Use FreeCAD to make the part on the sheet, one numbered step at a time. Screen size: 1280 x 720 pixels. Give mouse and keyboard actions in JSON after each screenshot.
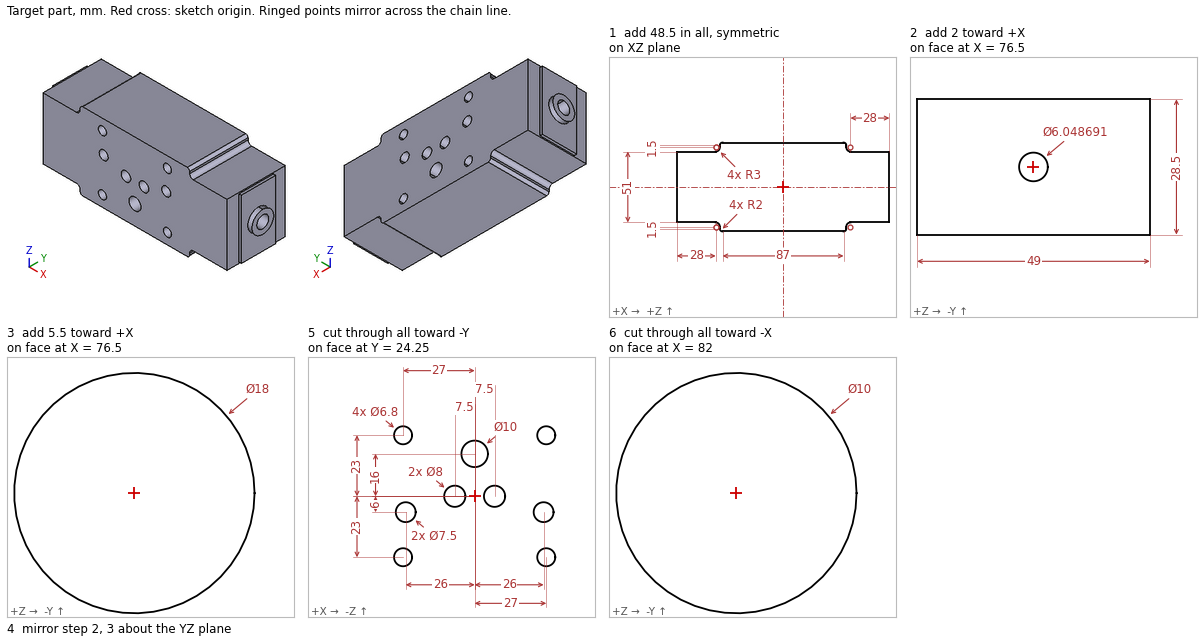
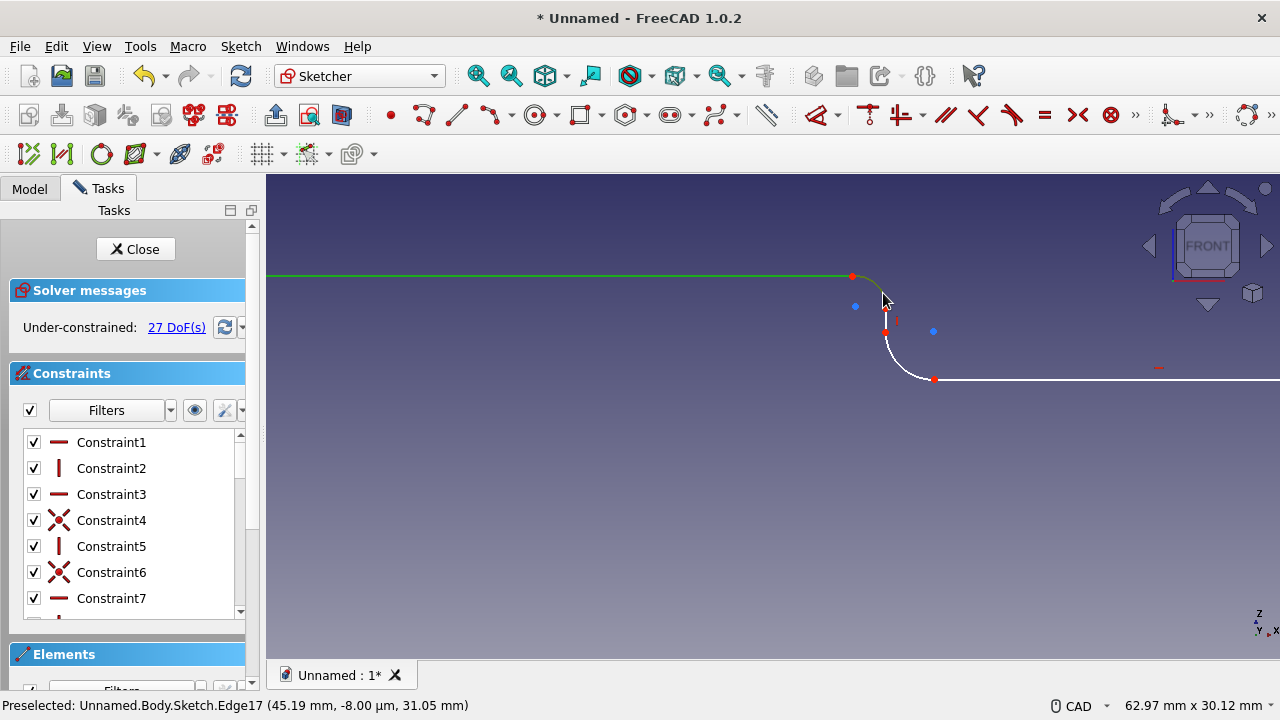
{"action": "left_click", "coordinate": [1012, 116]}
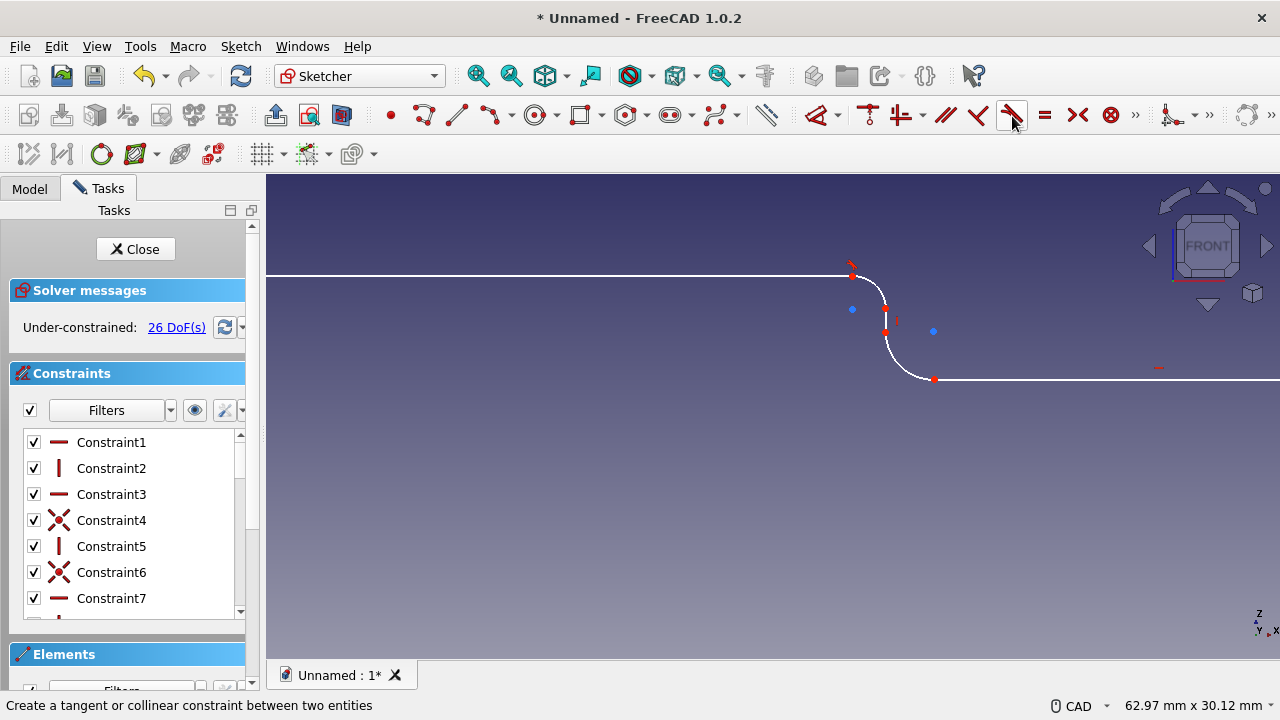
{"action": "scroll", "coordinate": [886, 318], "scroll_direction": "up", "scroll_amount": 2}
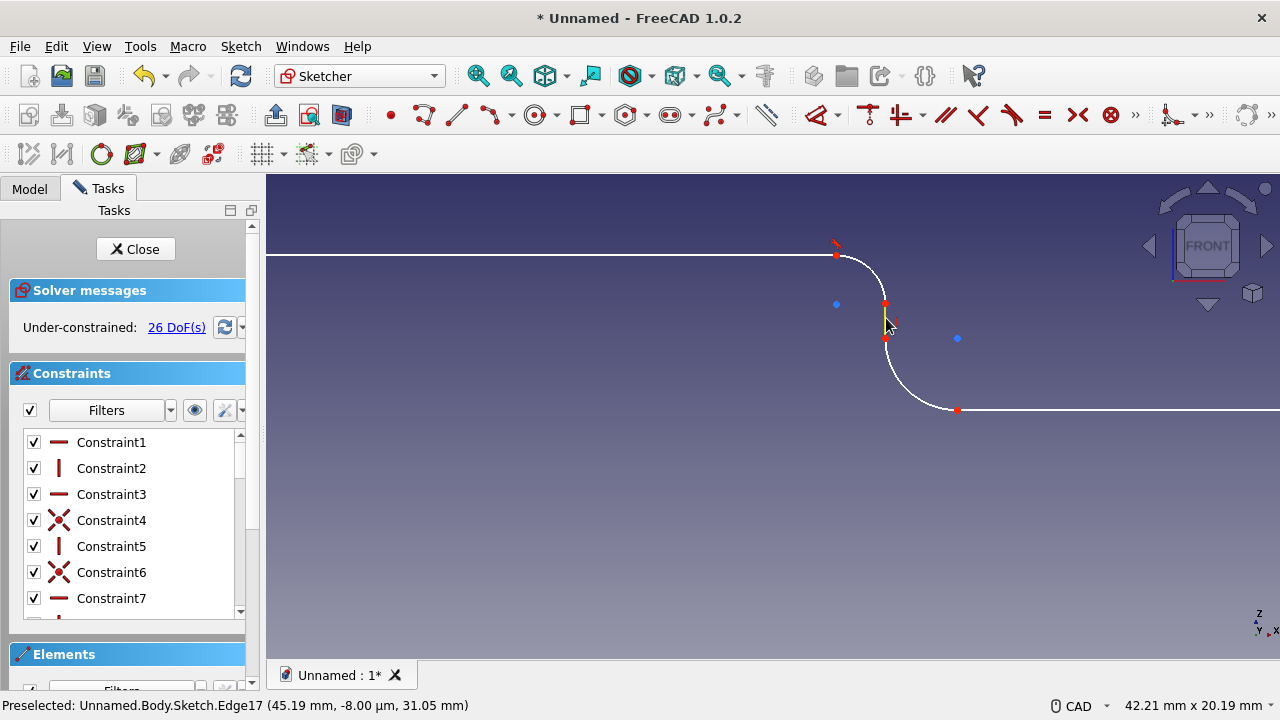
{"action": "left_click", "coordinate": [885, 318]}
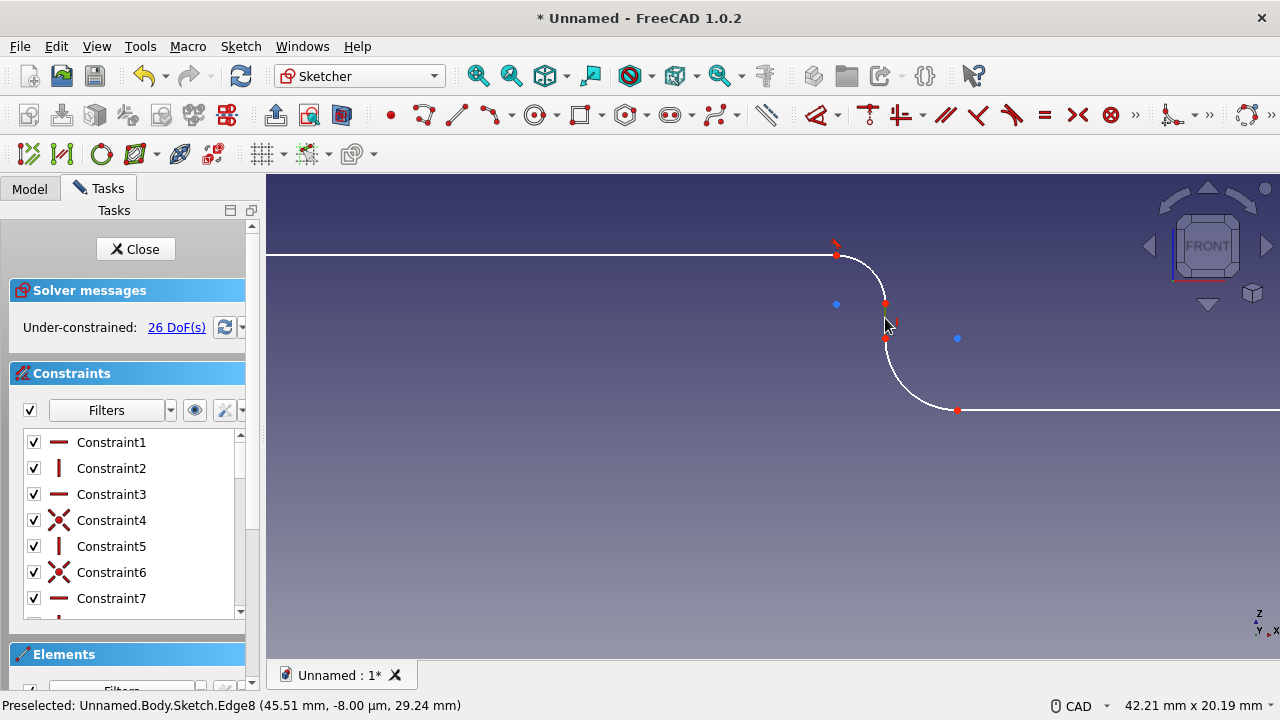
{"action": "left_click", "coordinate": [880, 282]}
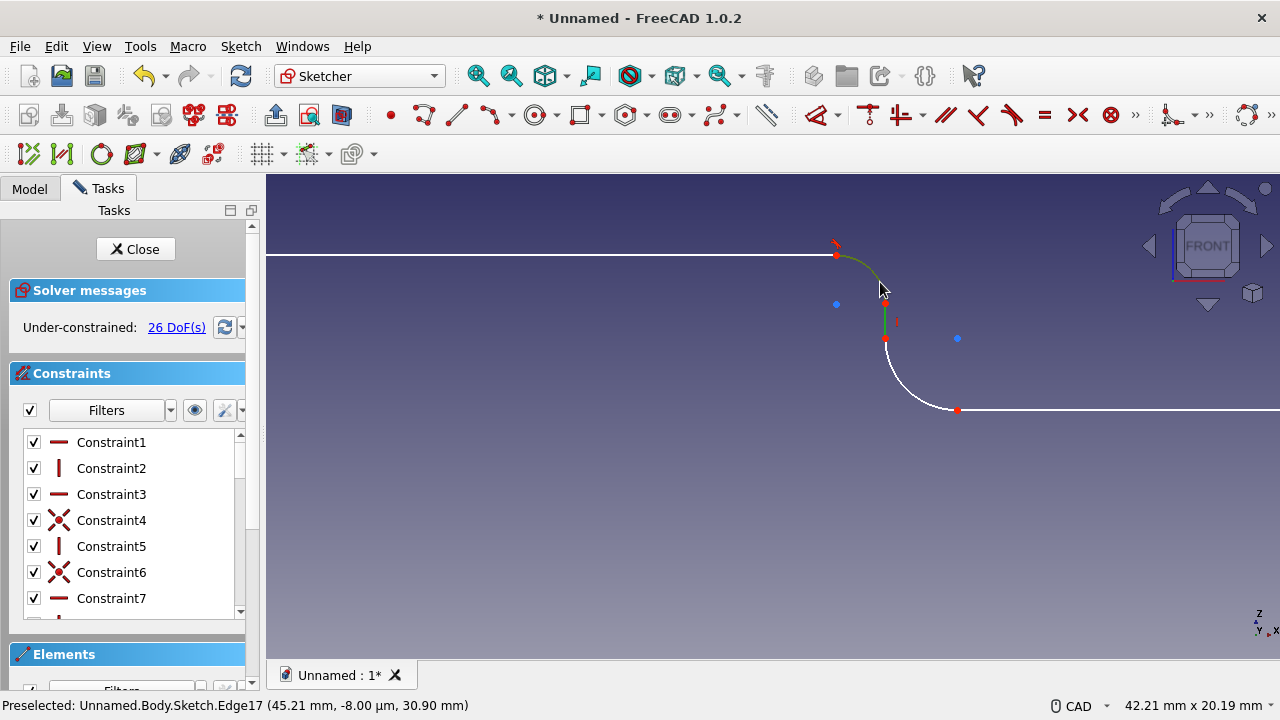
{"action": "left_click", "coordinate": [1012, 116]}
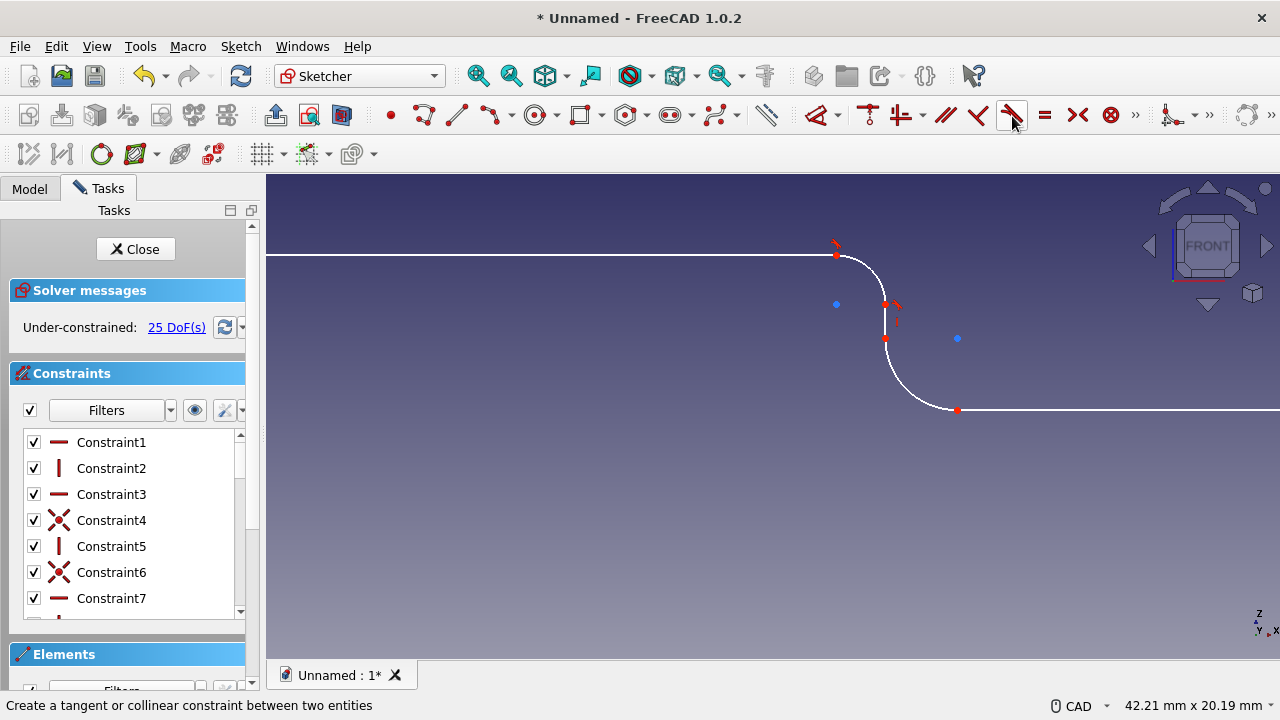
{"action": "scroll", "coordinate": [885, 315], "scroll_direction": "up", "scroll_amount": 2}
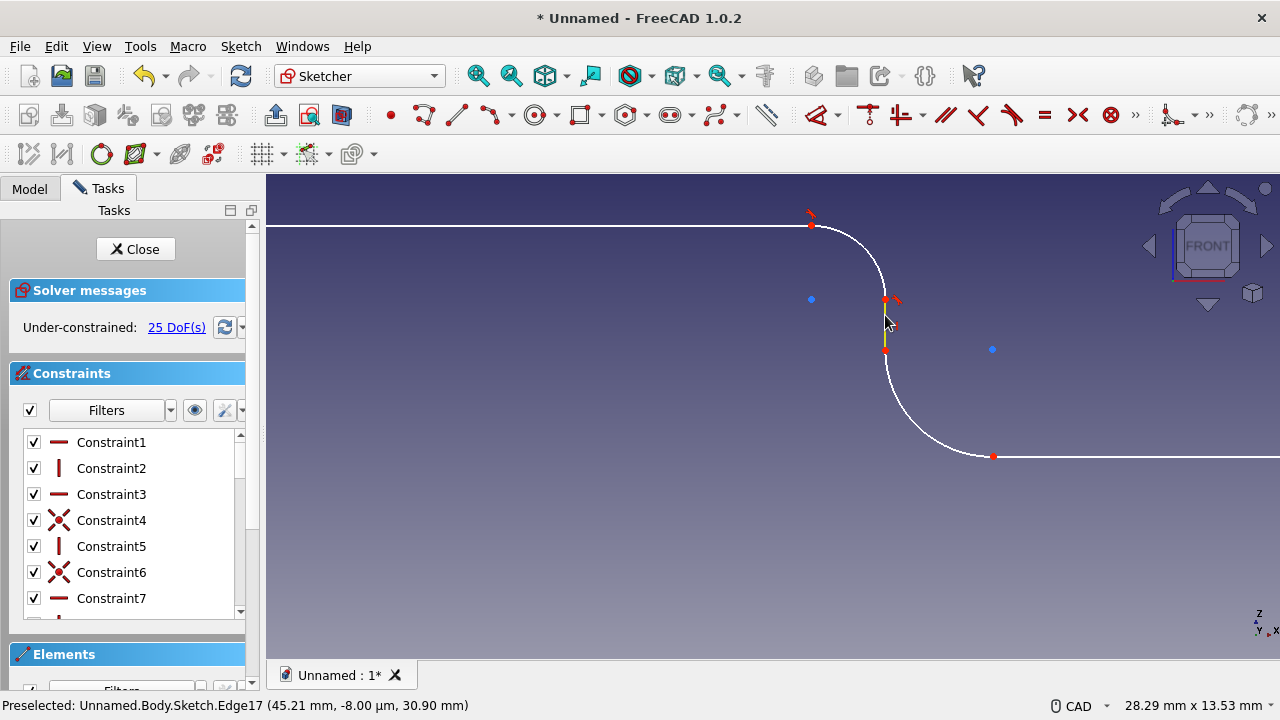
{"action": "left_click", "coordinate": [885, 315]}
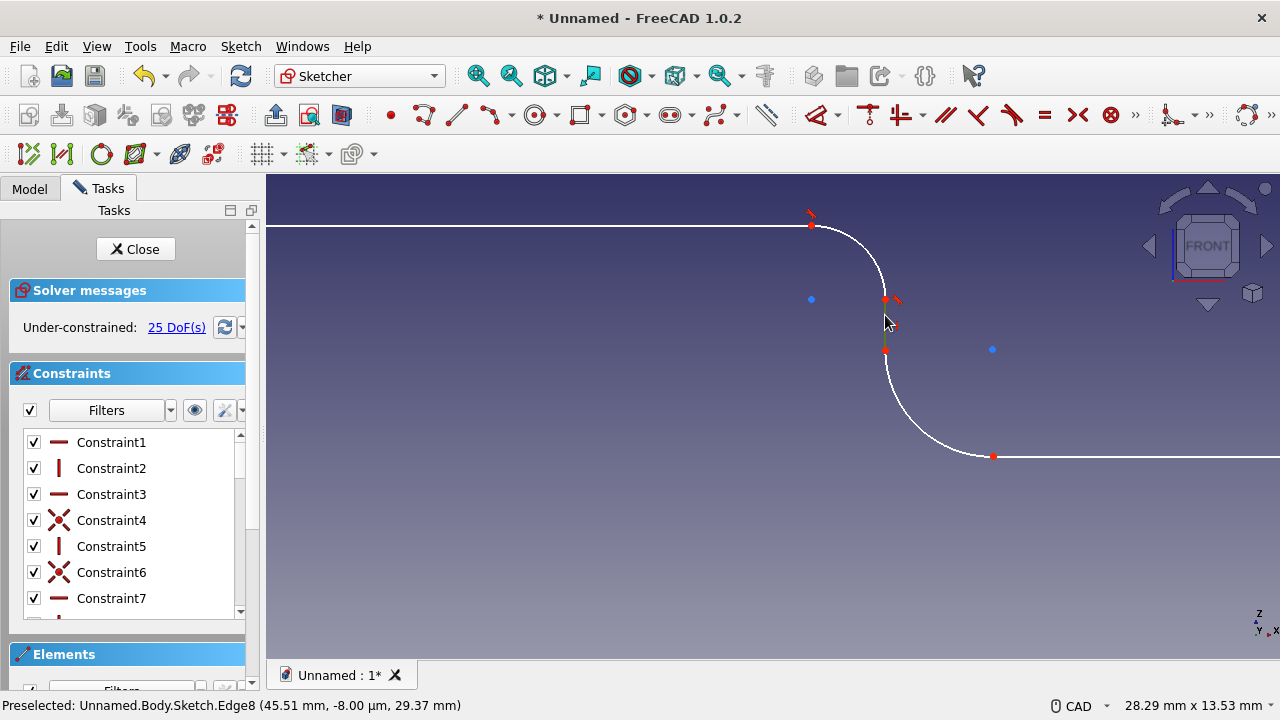
{"action": "scroll", "coordinate": [885, 298], "scroll_direction": "down", "scroll_amount": 11}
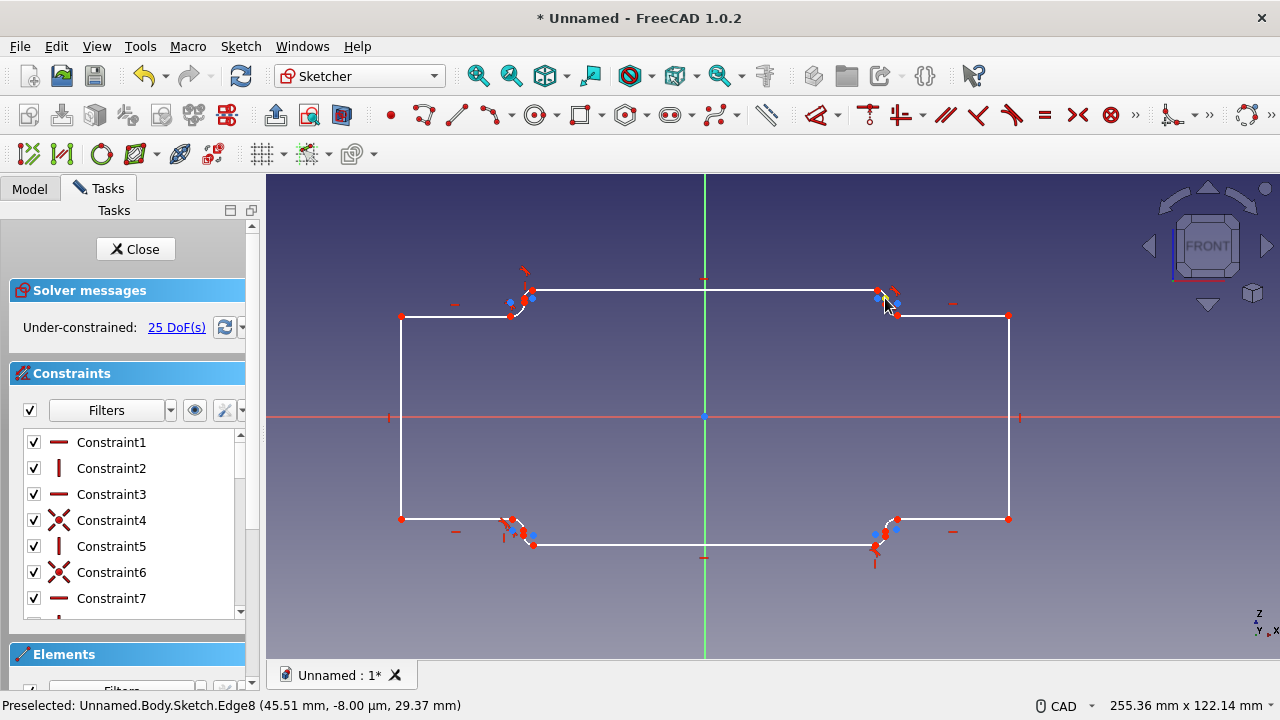
{"action": "scroll", "coordinate": [887, 309], "scroll_direction": "up", "scroll_amount": 5}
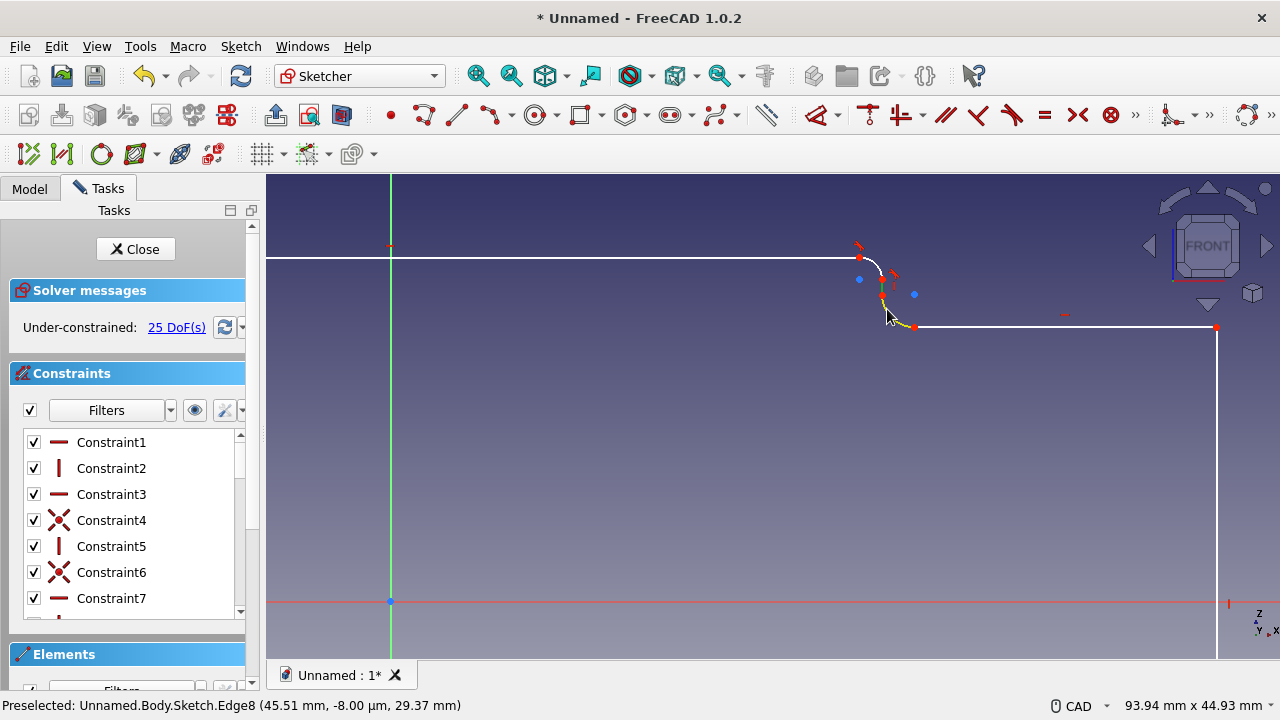
{"action": "left_click", "coordinate": [886, 310]}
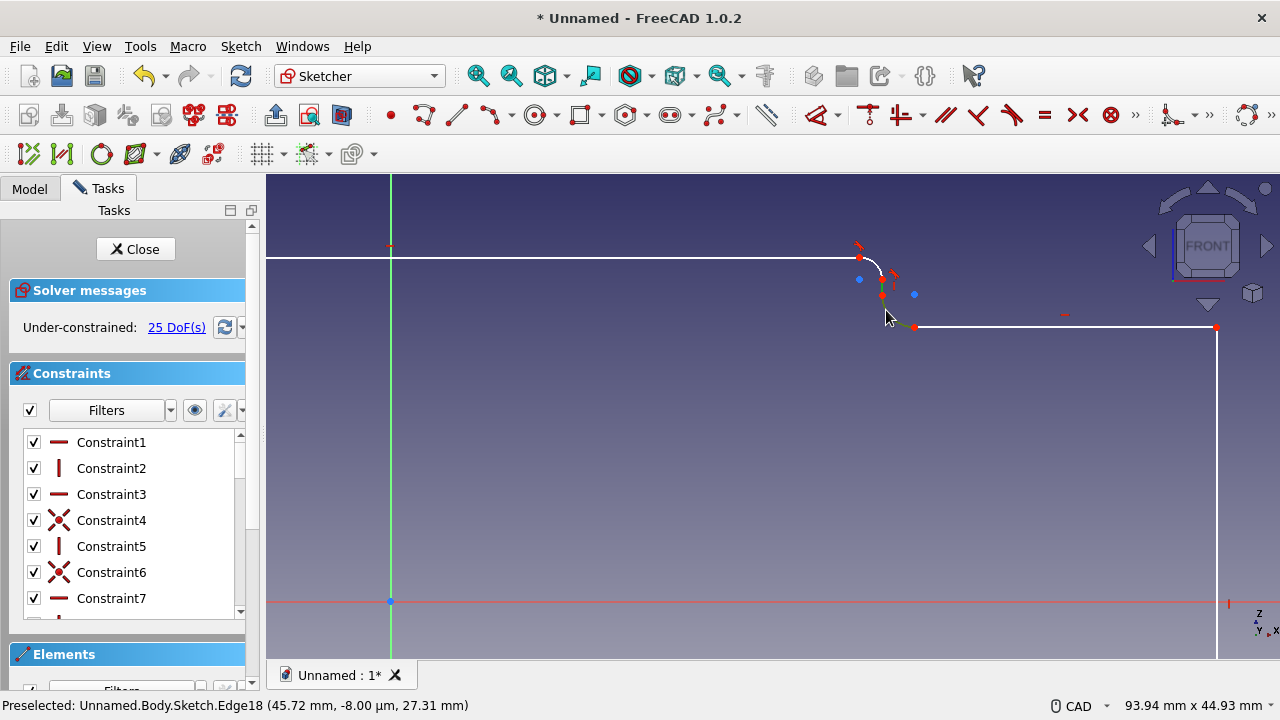
{"action": "left_click", "coordinate": [1012, 116]}